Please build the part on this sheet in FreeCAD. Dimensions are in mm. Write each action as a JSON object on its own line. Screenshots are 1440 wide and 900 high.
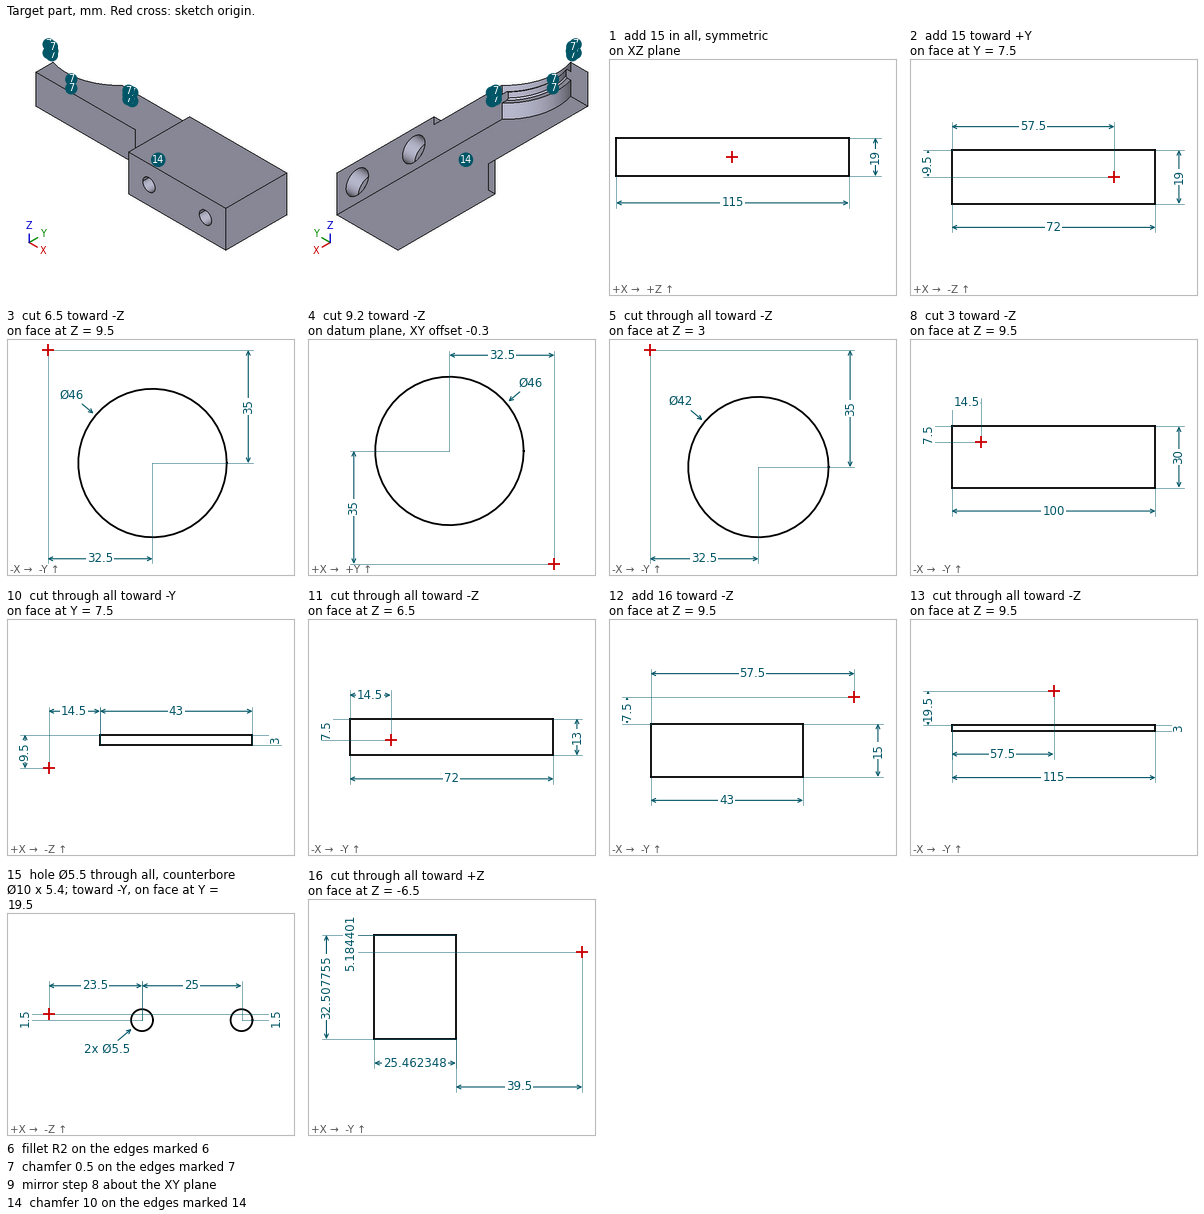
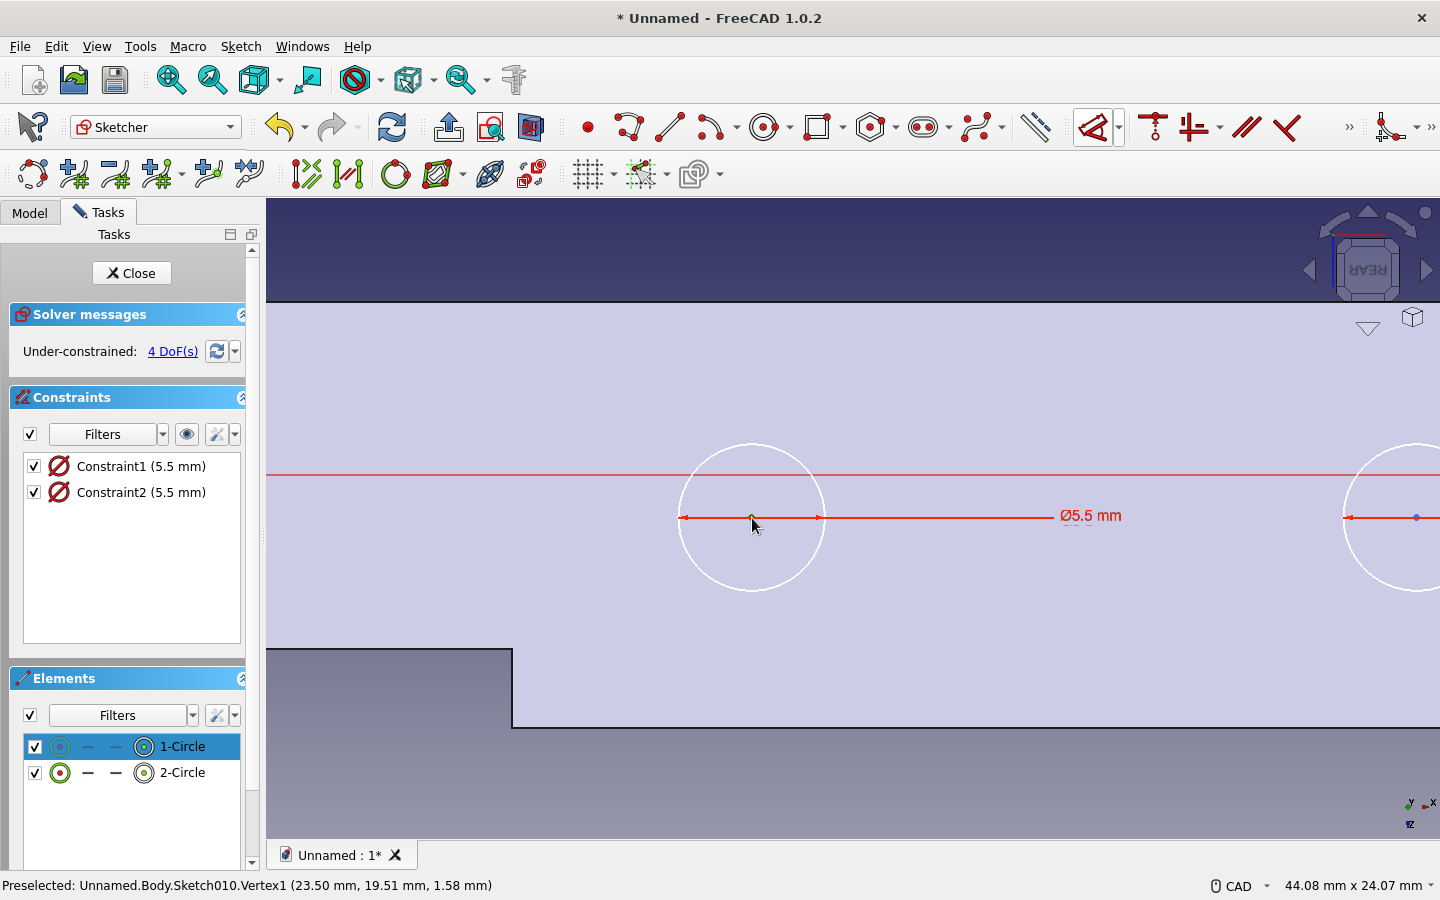
{"action": "left_click", "coordinate": [1118, 128]}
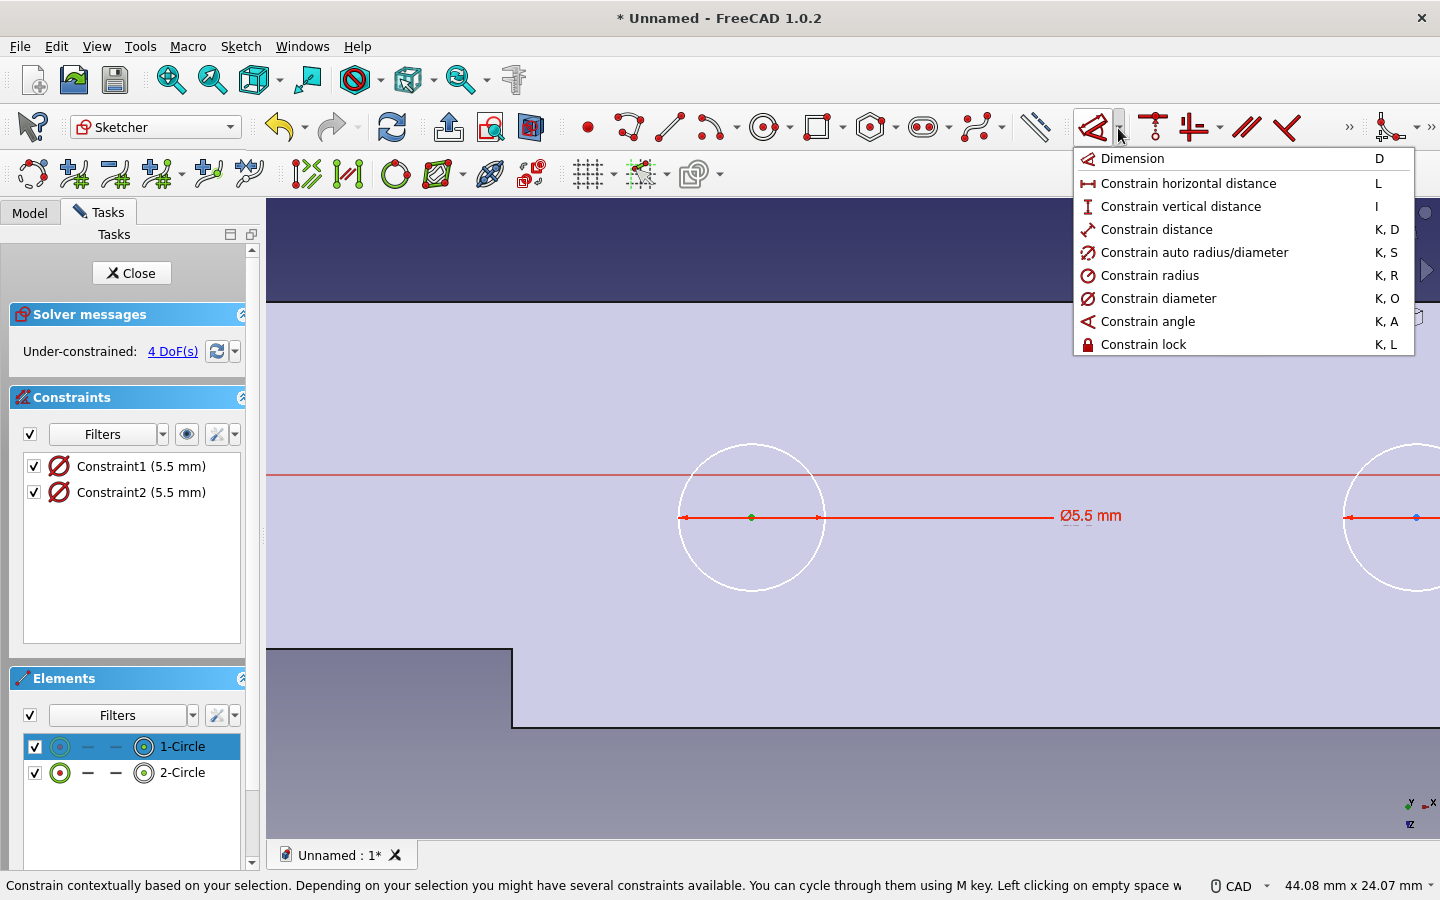
{"action": "left_click", "coordinate": [1244, 206]}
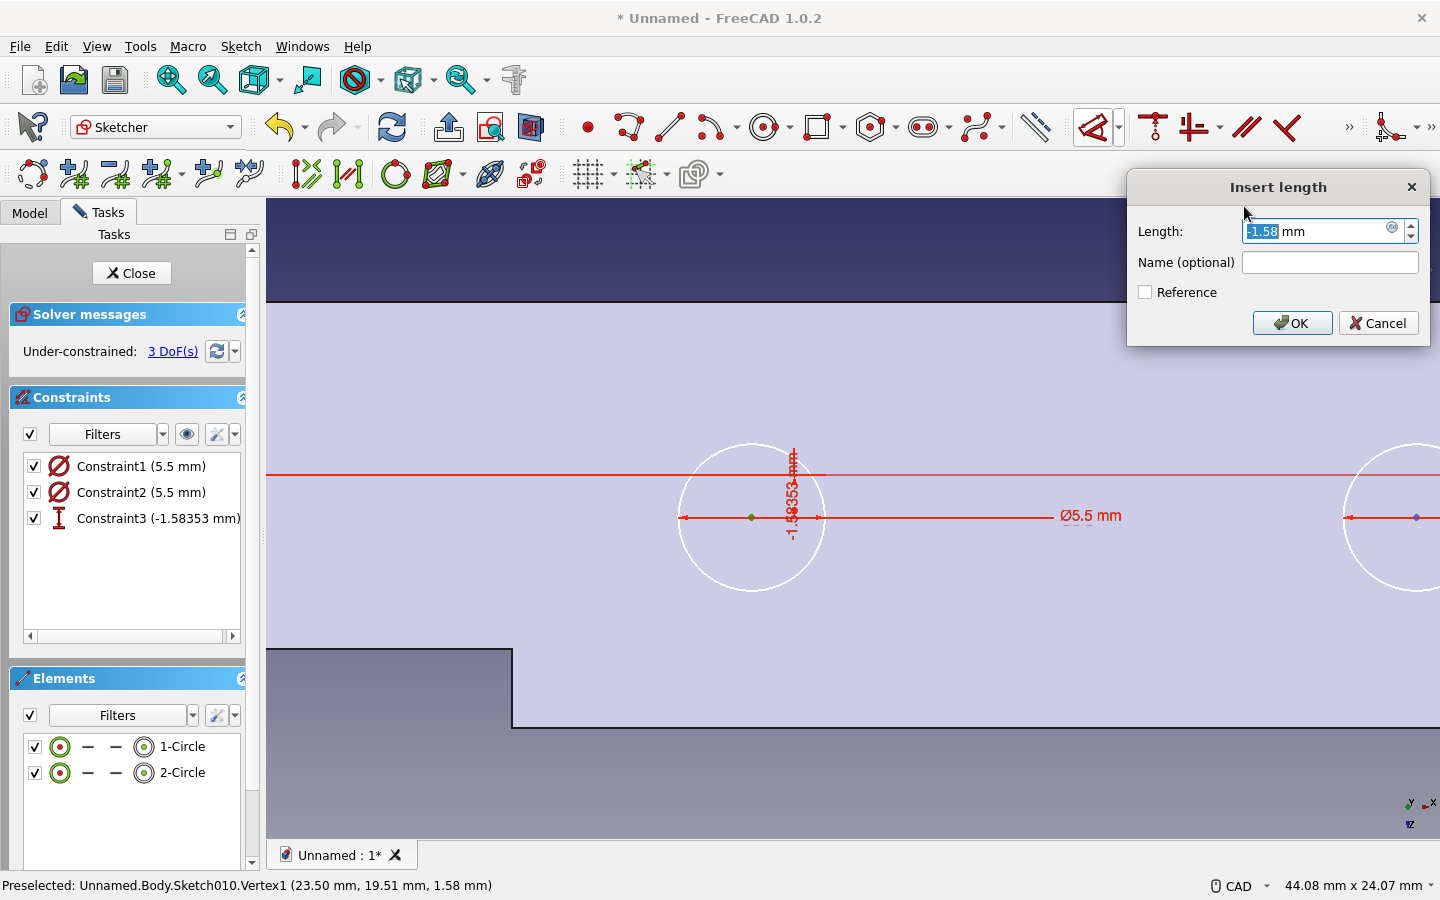
{"action": "type", "text": "-1.5"}
{"action": "key", "text": "Return"}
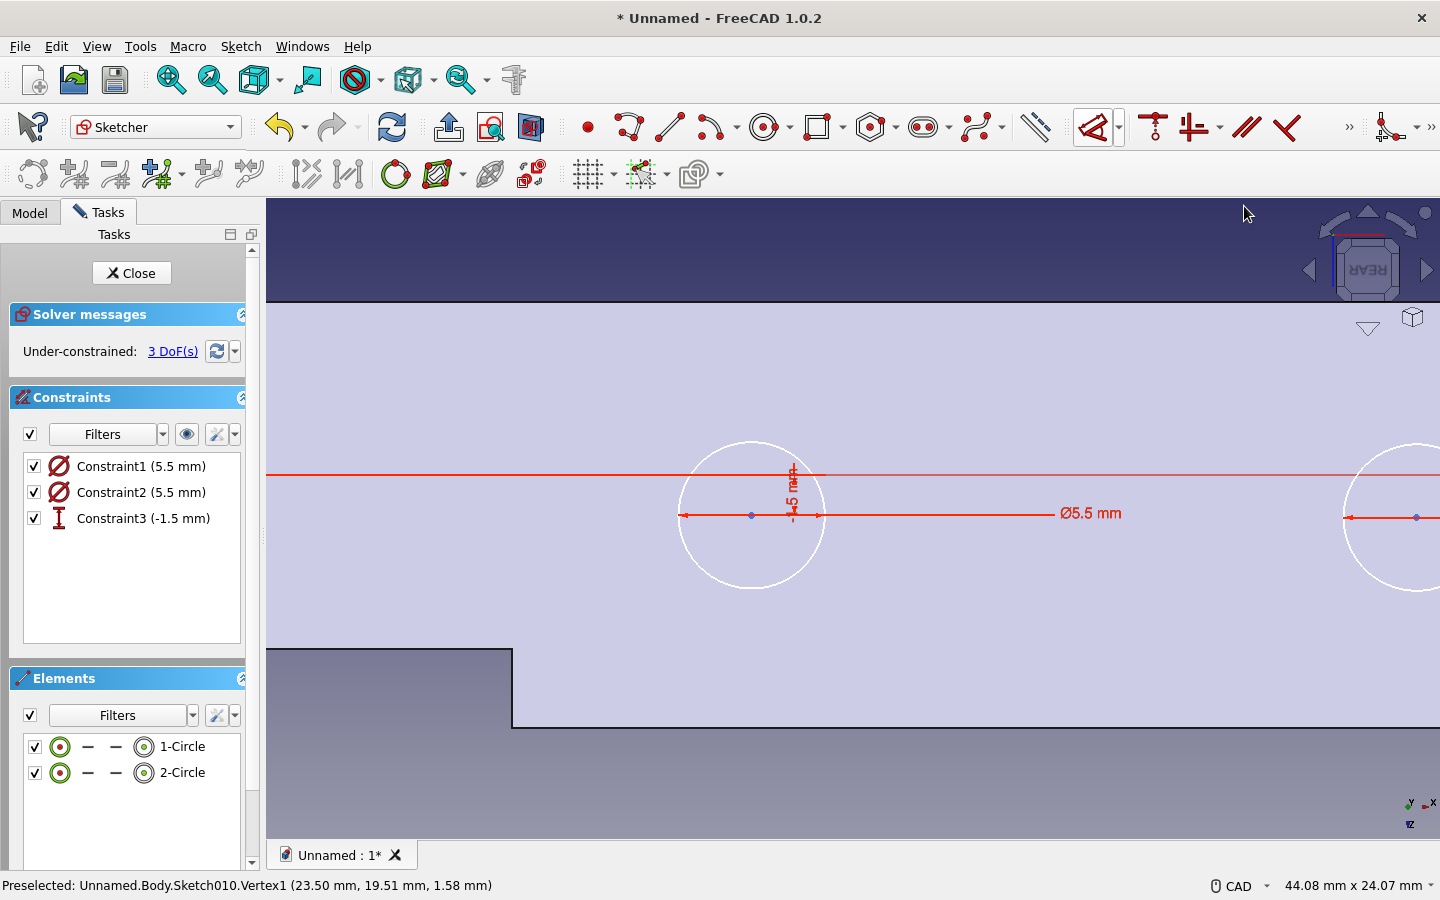
{"action": "scroll", "coordinate": [756, 522], "scroll_direction": "down", "scroll_amount": 3}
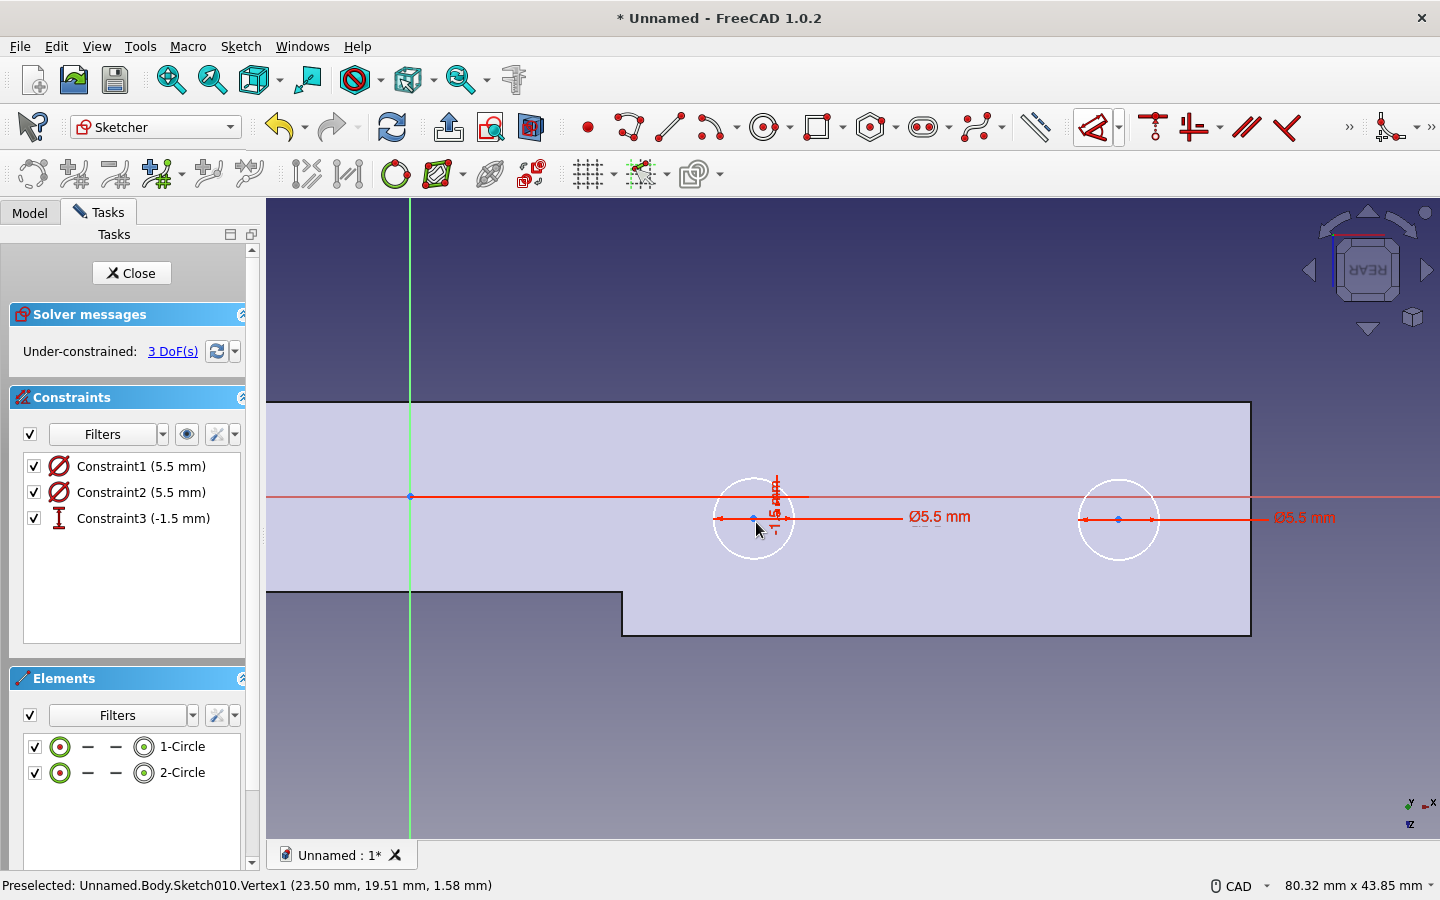
{"action": "scroll", "coordinate": [1119, 520], "scroll_direction": "up", "scroll_amount": 3}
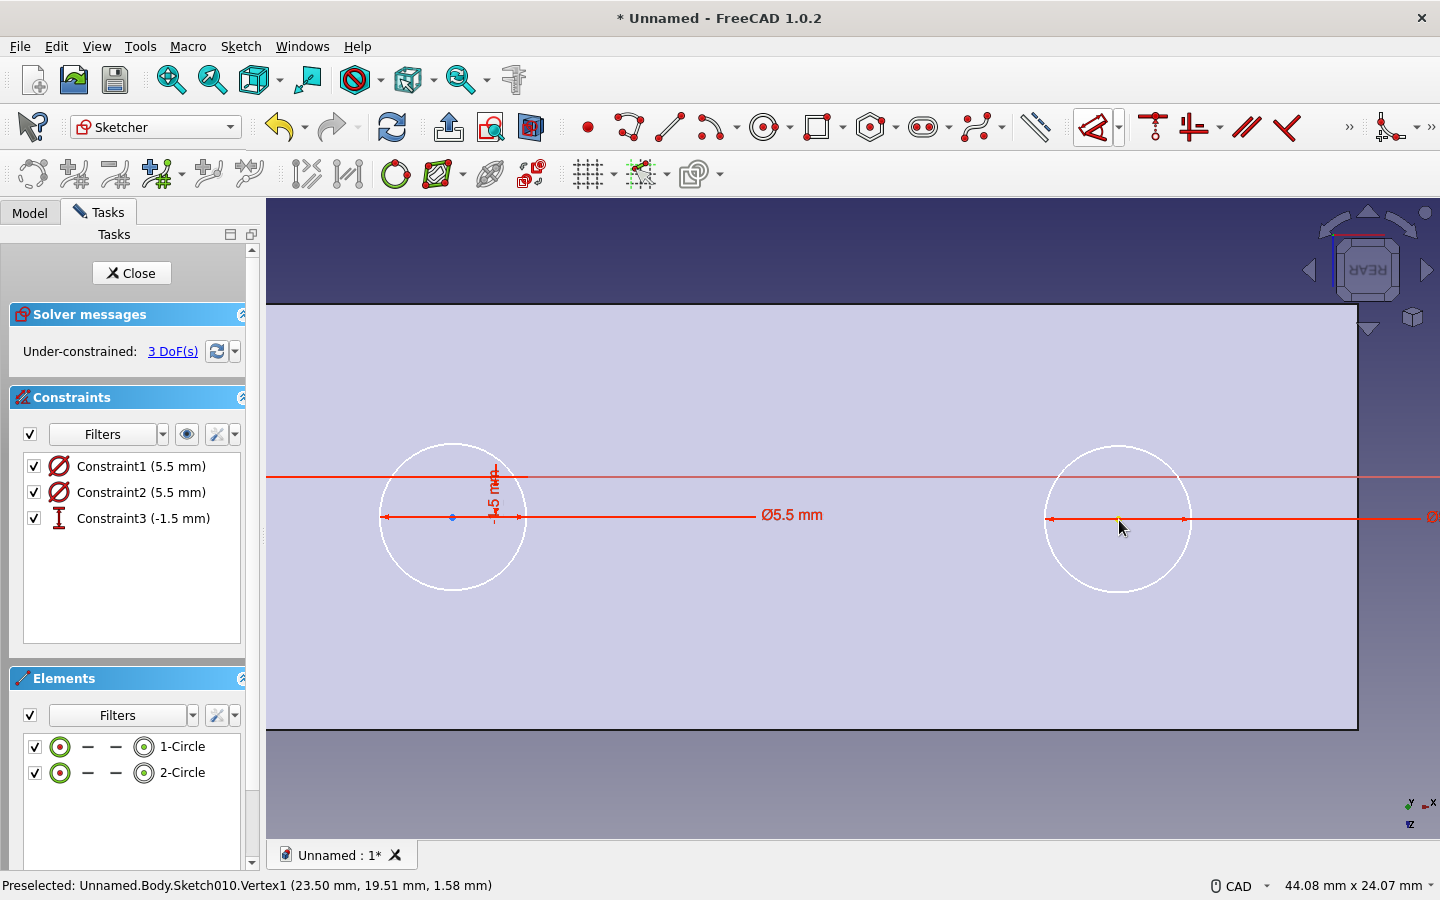
{"action": "left_click", "coordinate": [1118, 519]}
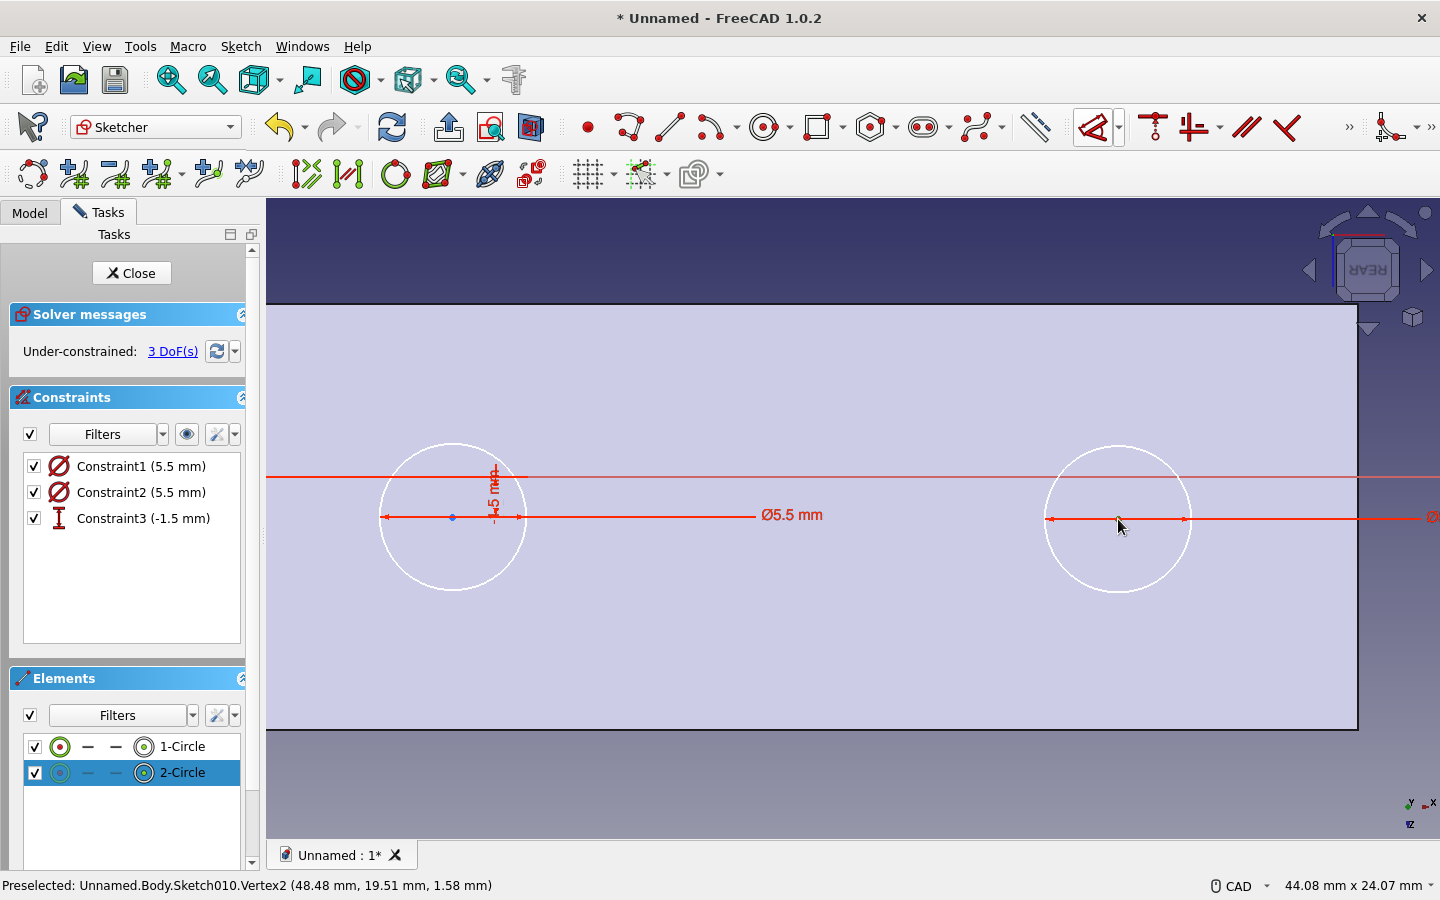
{"action": "left_click", "coordinate": [1118, 128]}